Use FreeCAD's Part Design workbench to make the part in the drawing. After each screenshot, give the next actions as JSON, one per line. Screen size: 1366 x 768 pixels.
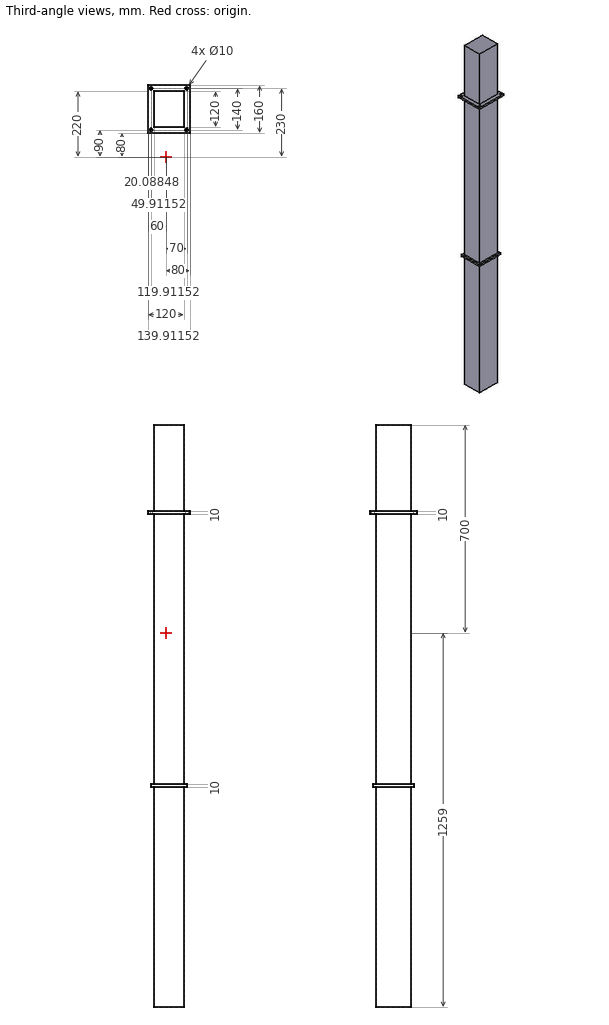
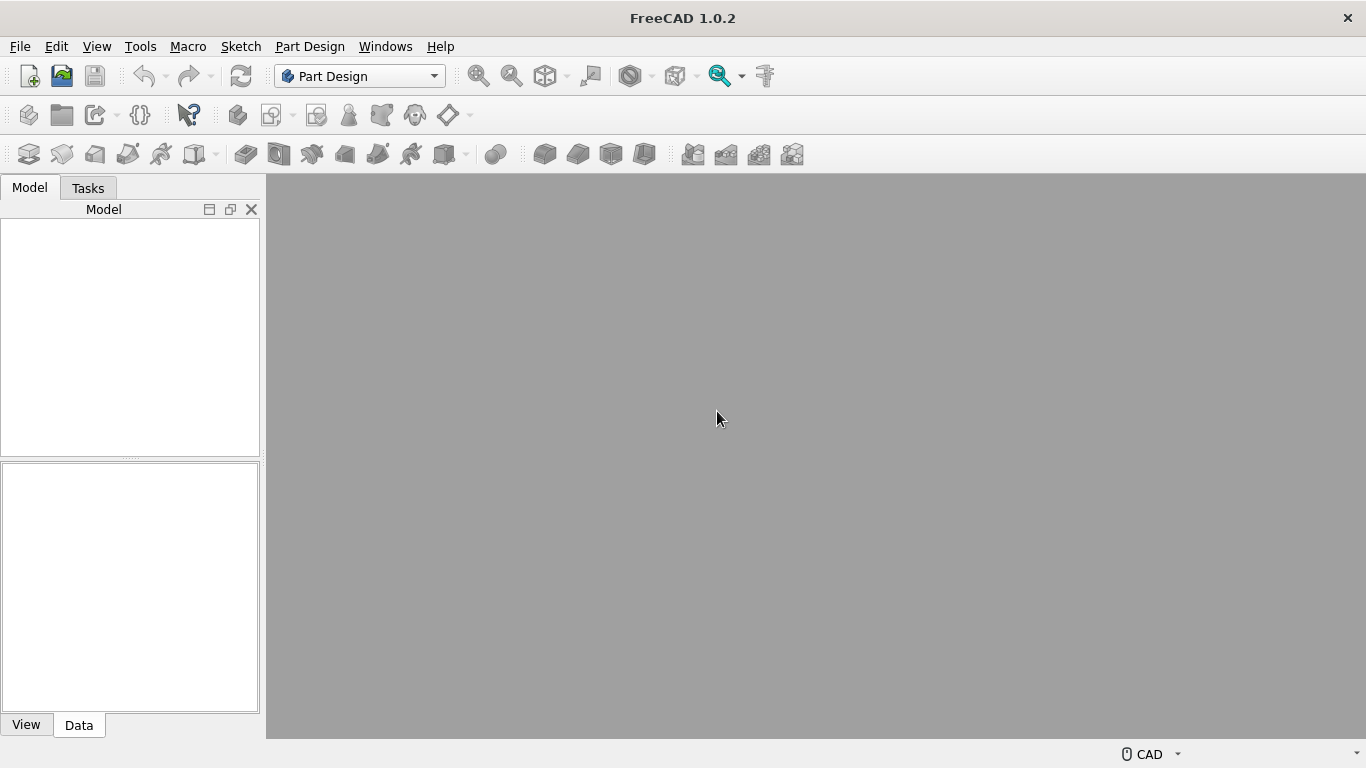
{"action": "left_click", "coordinate": [29, 76]}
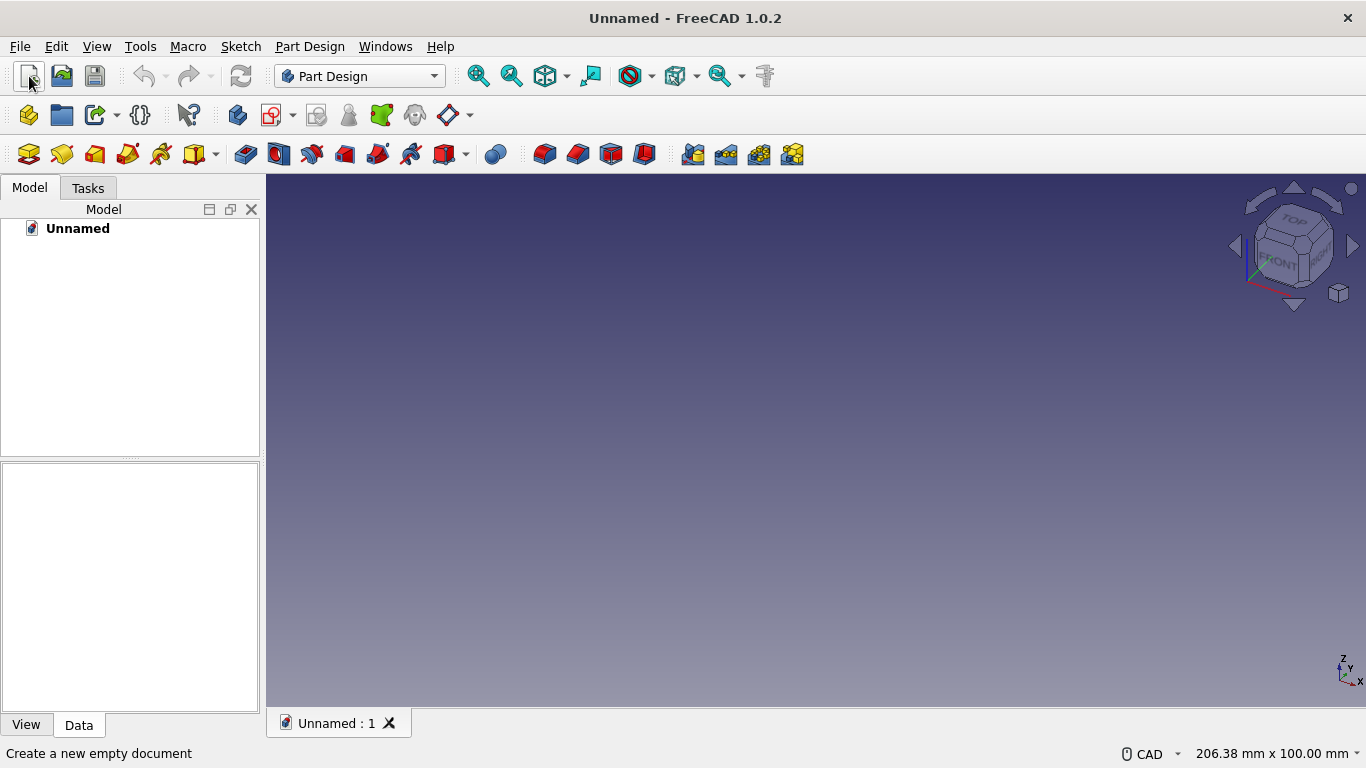
{"action": "left_click", "coordinate": [270, 116]}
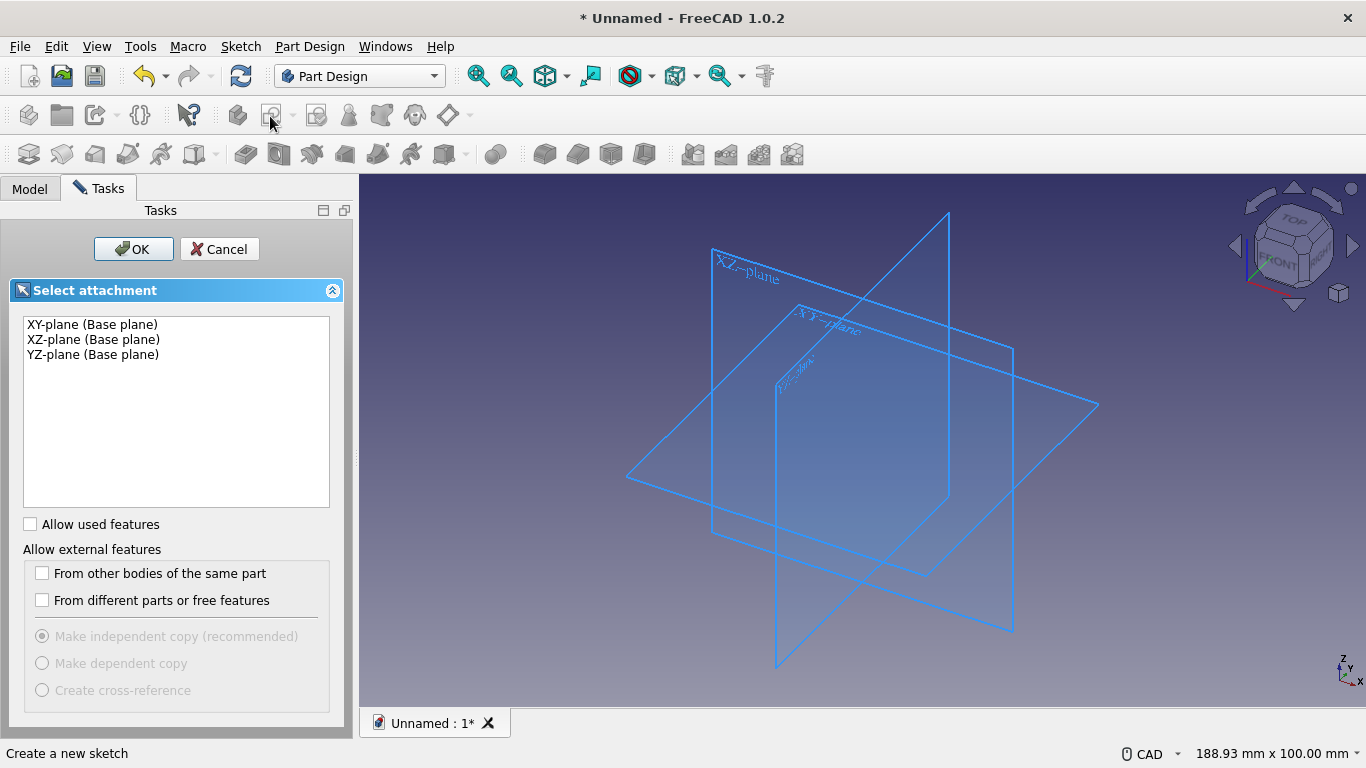
{"action": "left_click", "coordinate": [84, 324]}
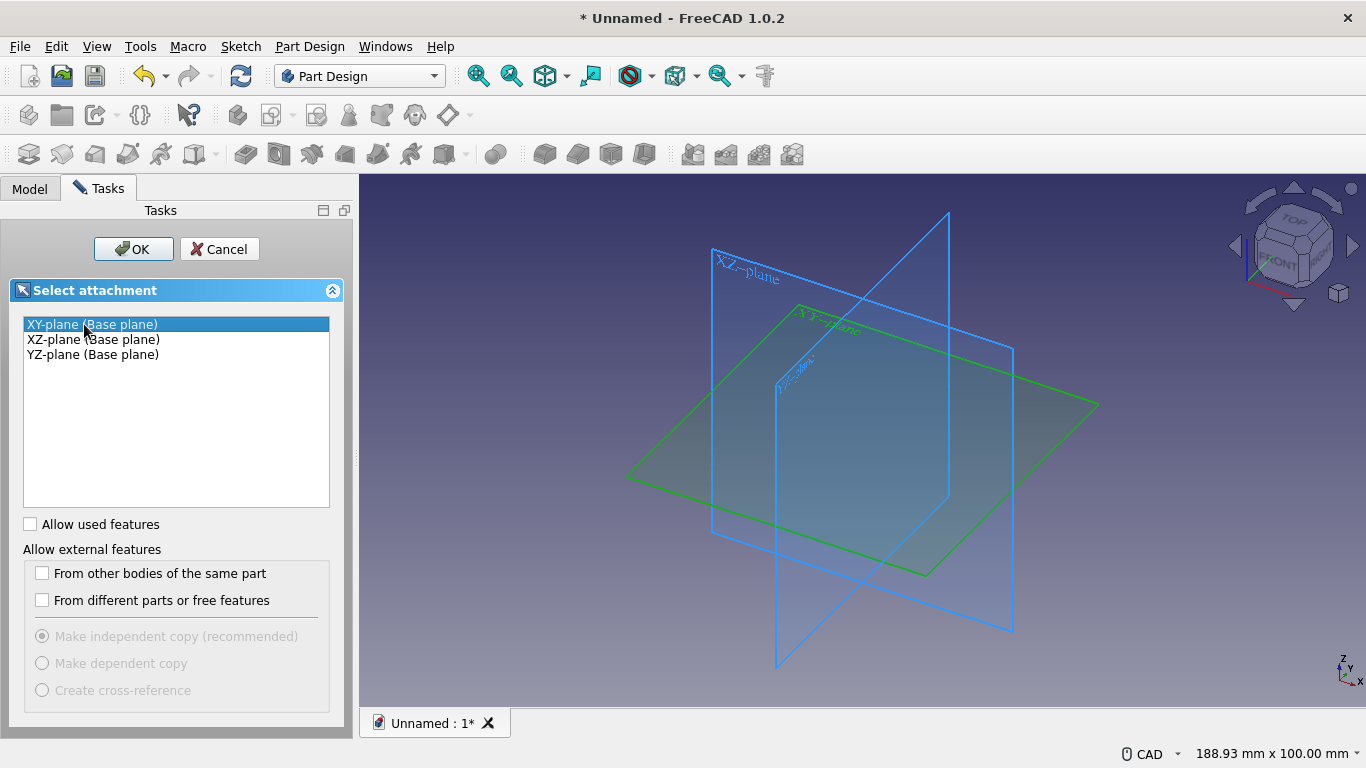
{"action": "left_click", "coordinate": [134, 249]}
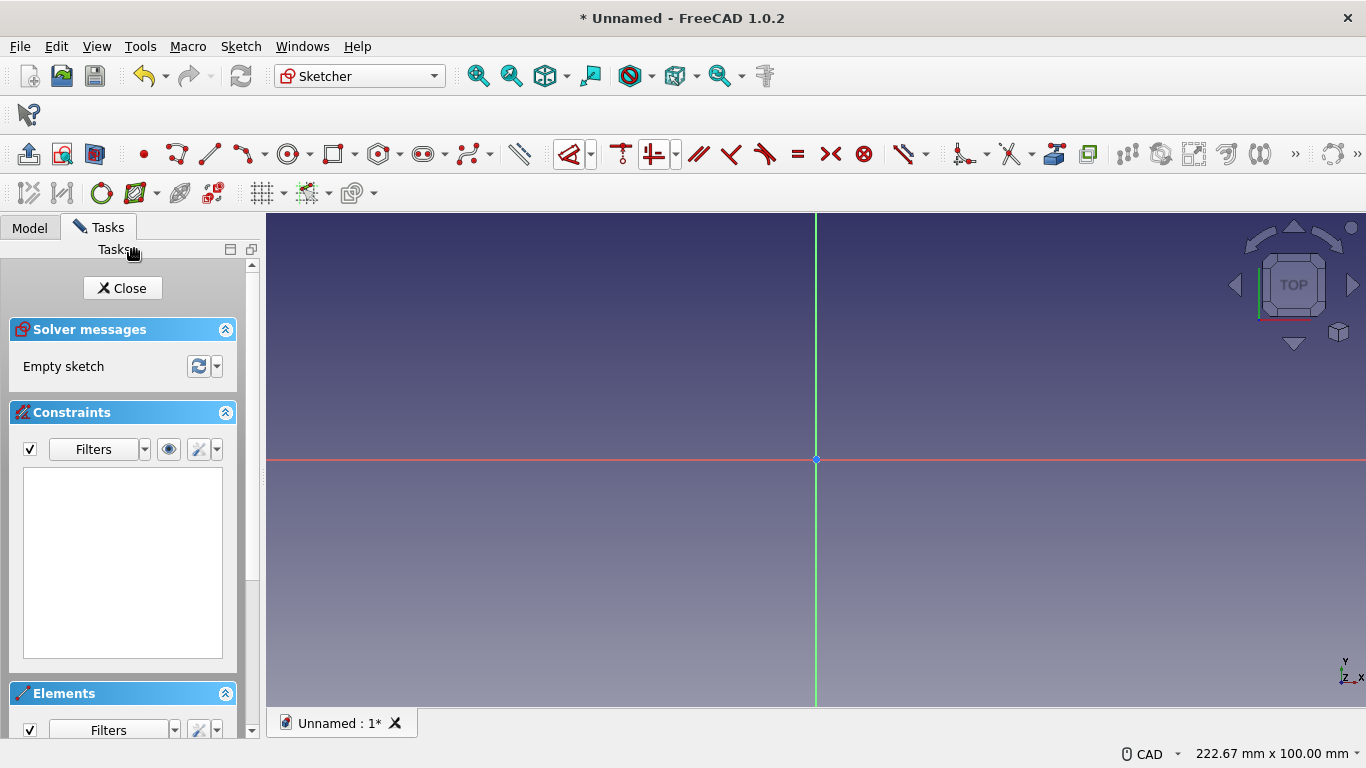
{"action": "scroll", "coordinate": [718, 679], "scroll_direction": "down", "scroll_amount": 6}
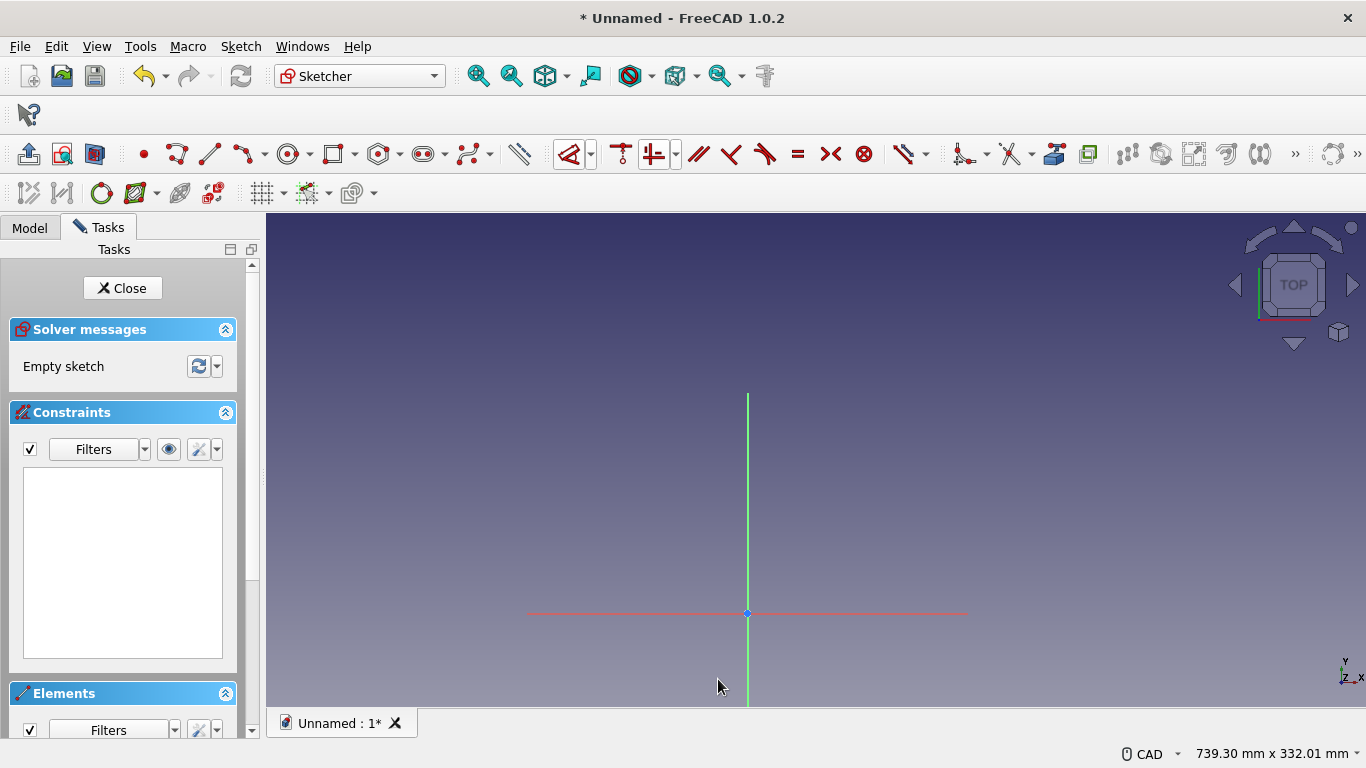
{"action": "key", "text": "g r"}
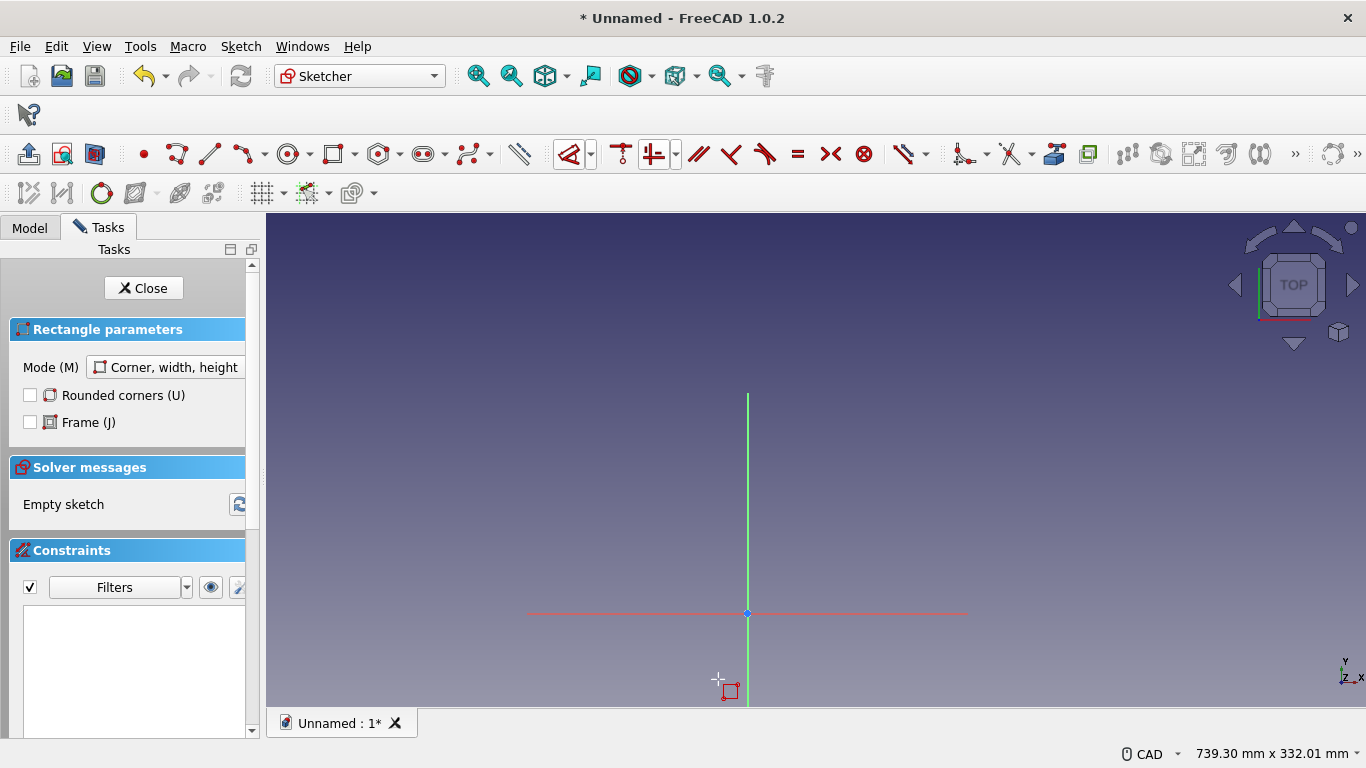
{"action": "left_click", "coordinate": [659, 286]}
{"action": "mouse_move", "coordinate": [837, 465]}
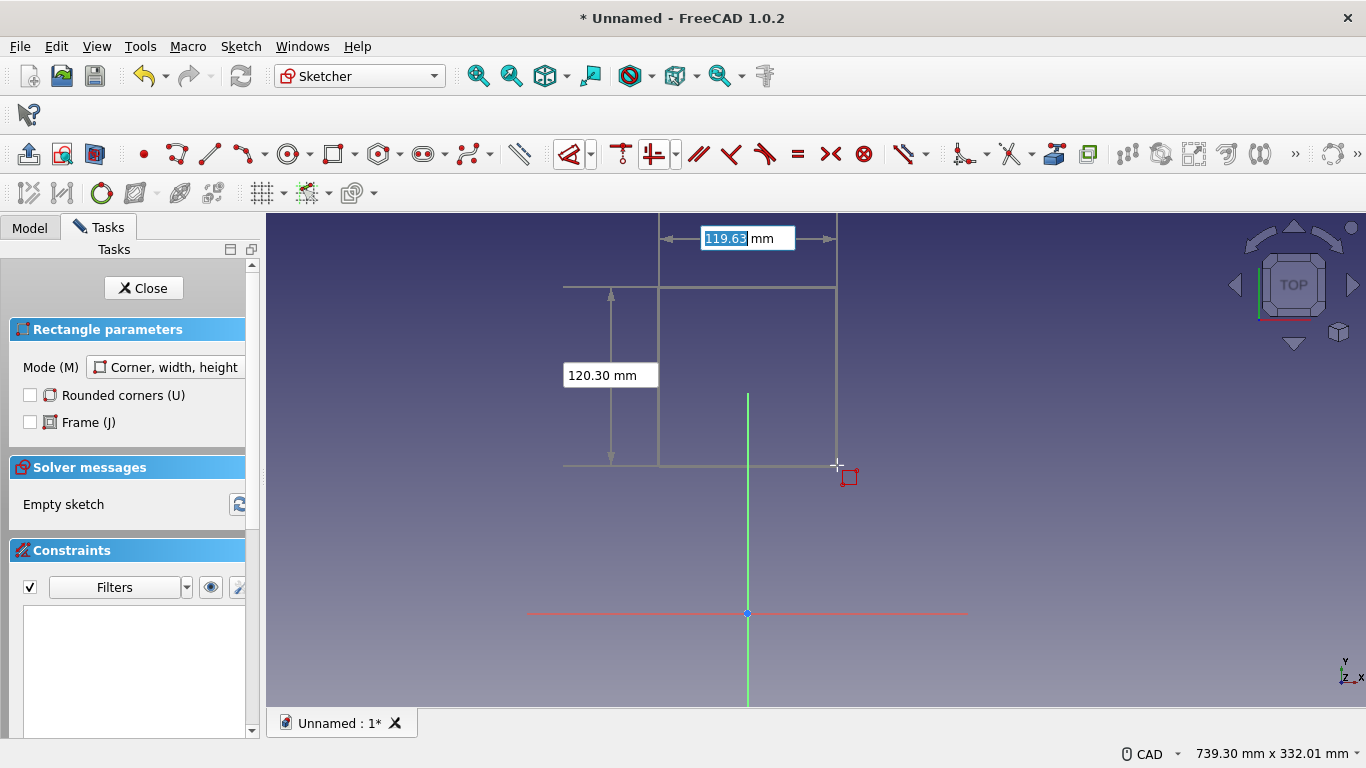
{"action": "type", "text": "120"}
{"action": "key", "text": "Tab"}
{"action": "type", "text": "120"}
{"action": "key", "text": "Return"}
{"action": "key", "text": "Escape"}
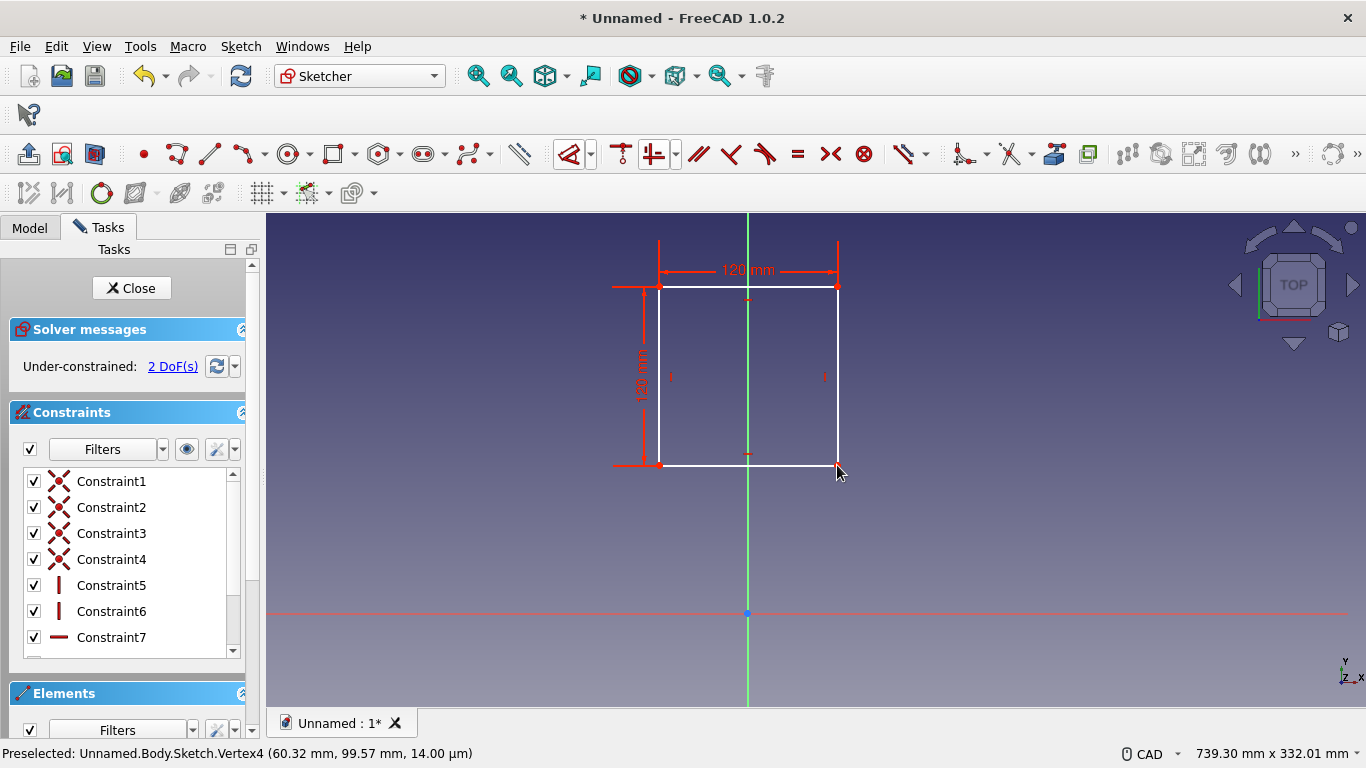
{"action": "left_click", "coordinate": [568, 154]}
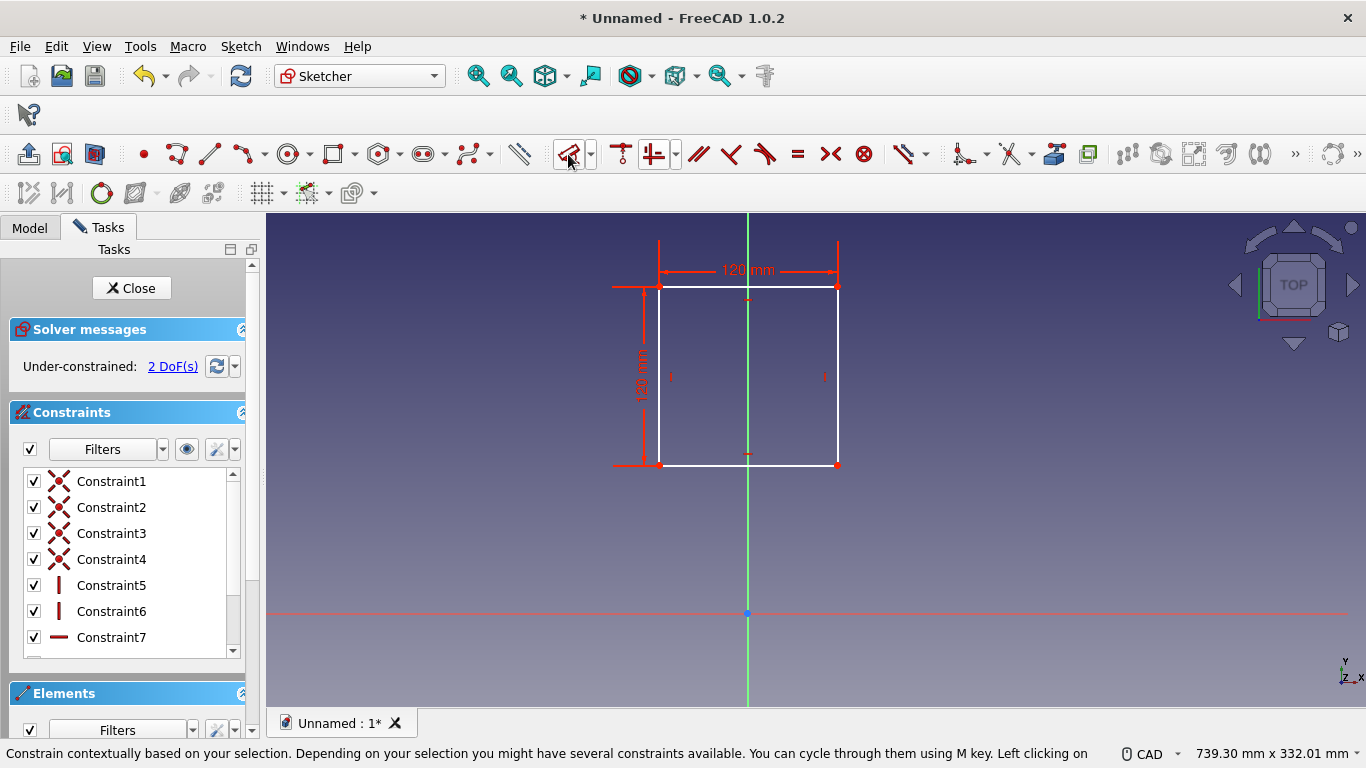
{"action": "left_click", "coordinate": [659, 287]}
{"action": "left_click", "coordinate": [703, 648]}